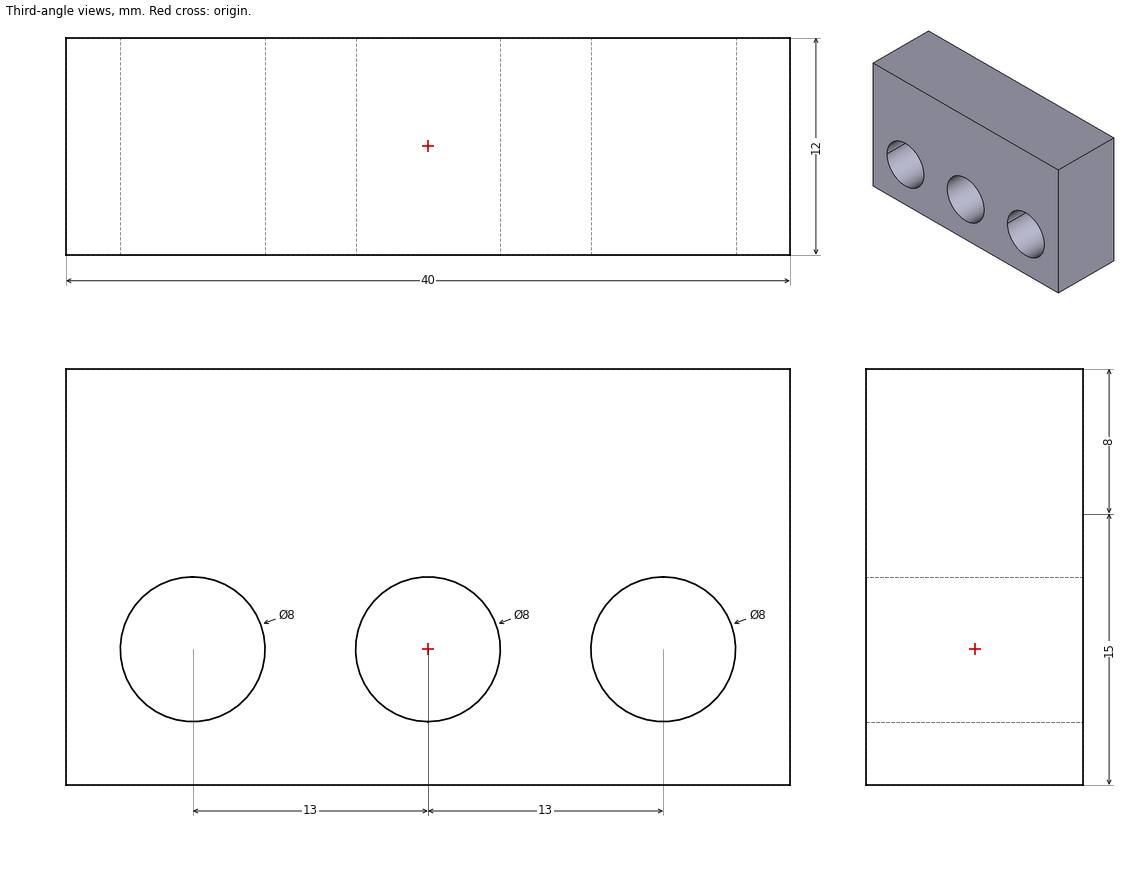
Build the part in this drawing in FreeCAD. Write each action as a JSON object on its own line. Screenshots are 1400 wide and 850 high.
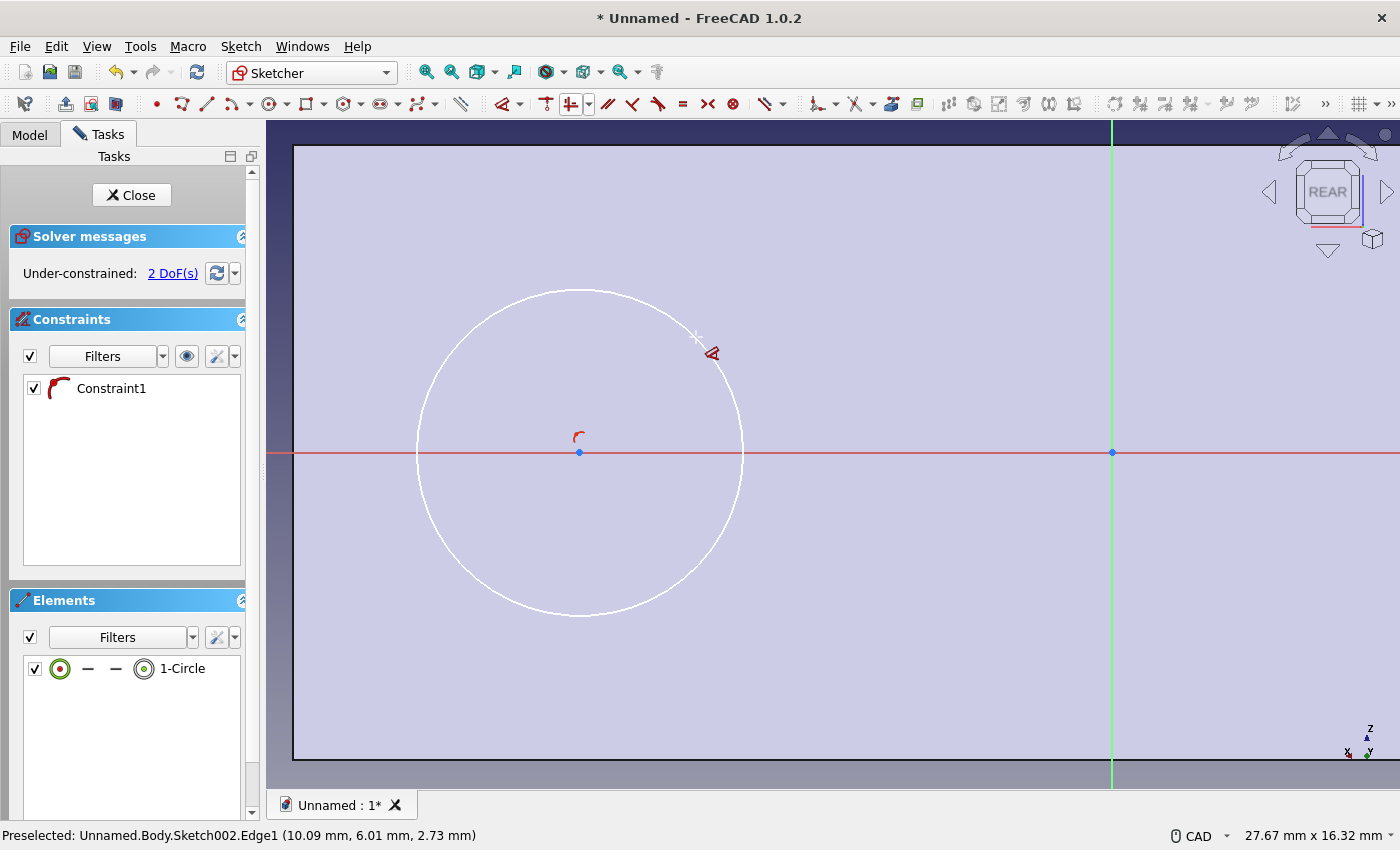
{"action": "left_click", "coordinate": [695, 337]}
{"action": "left_click", "coordinate": [718, 314]}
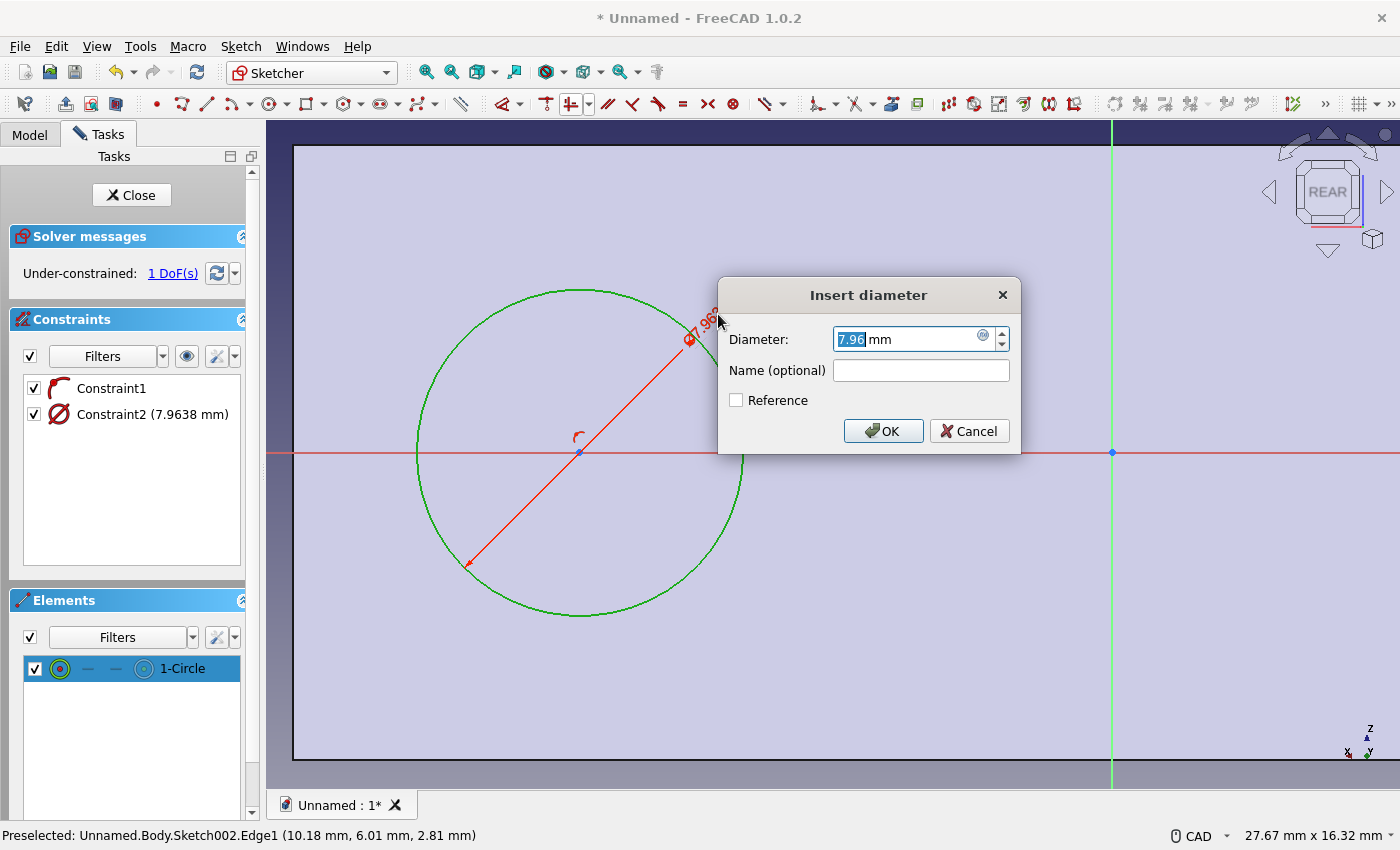
{"action": "type", "text": "8"}
{"action": "key", "text": "Return"}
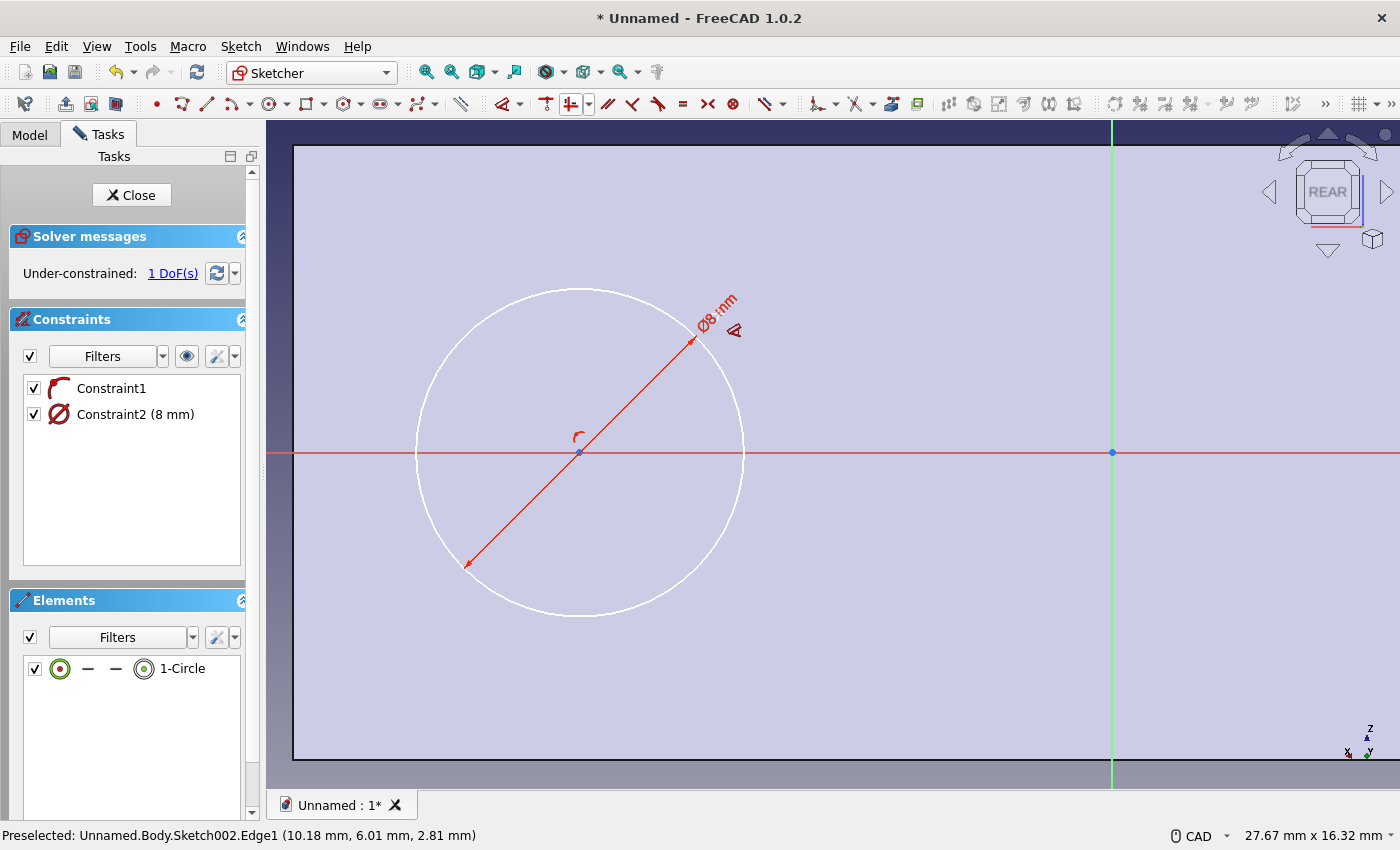
{"action": "left_click", "coordinate": [580, 453]}
{"action": "left_click", "coordinate": [846, 487]}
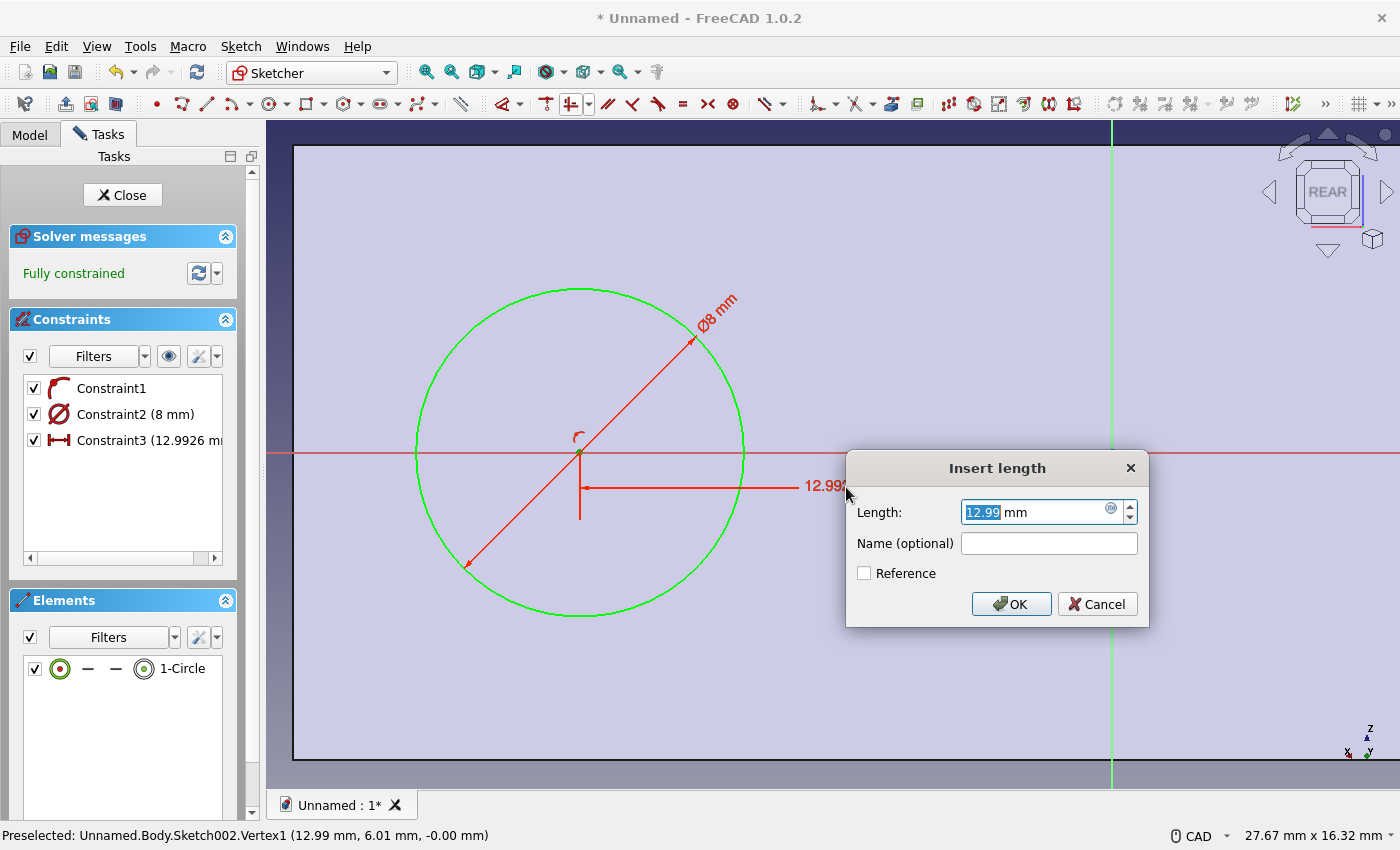
{"action": "type", "text": "13"}
{"action": "key", "text": "Return"}
{"action": "key", "text": "Escape"}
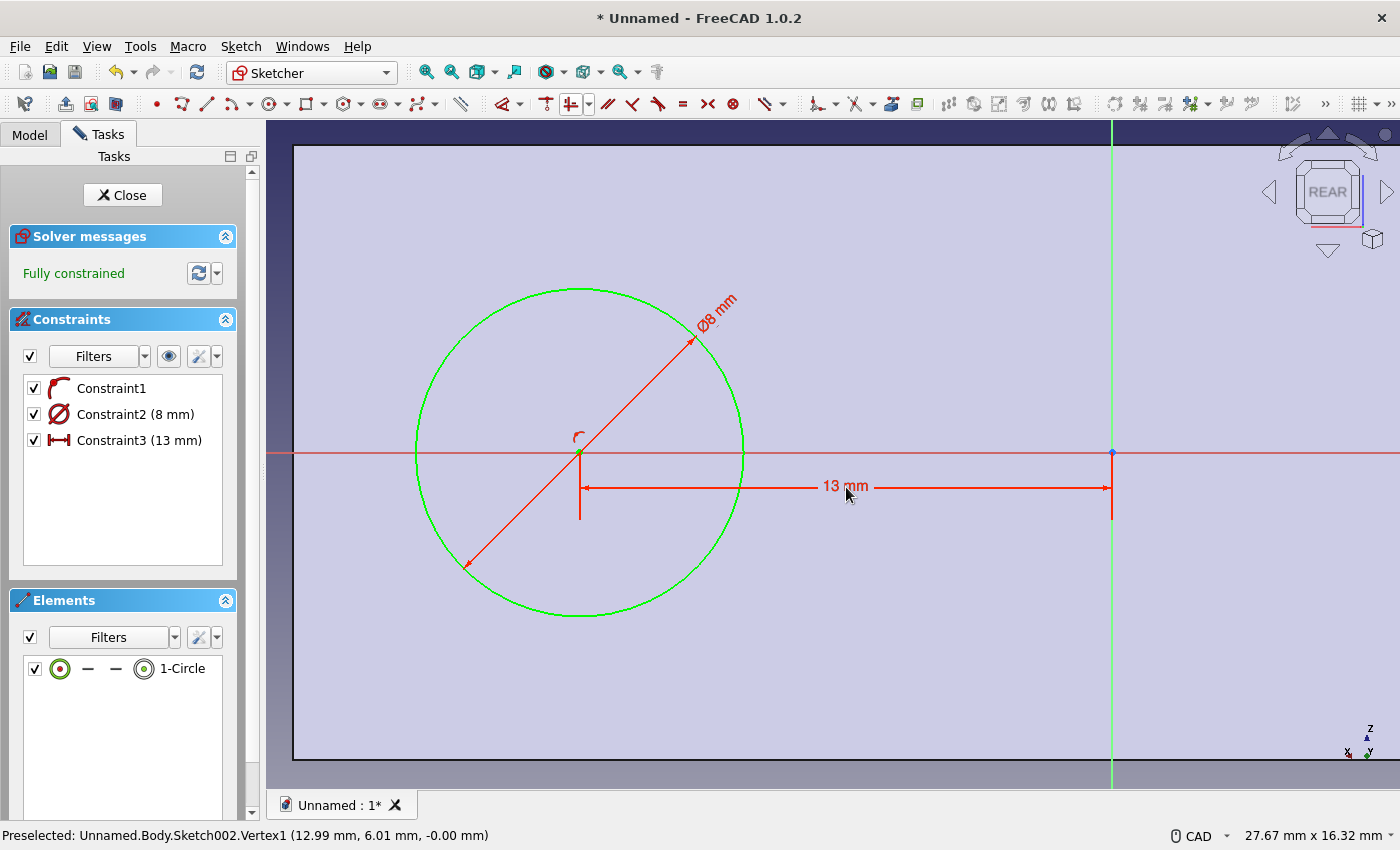
{"action": "left_click", "coordinate": [123, 195]}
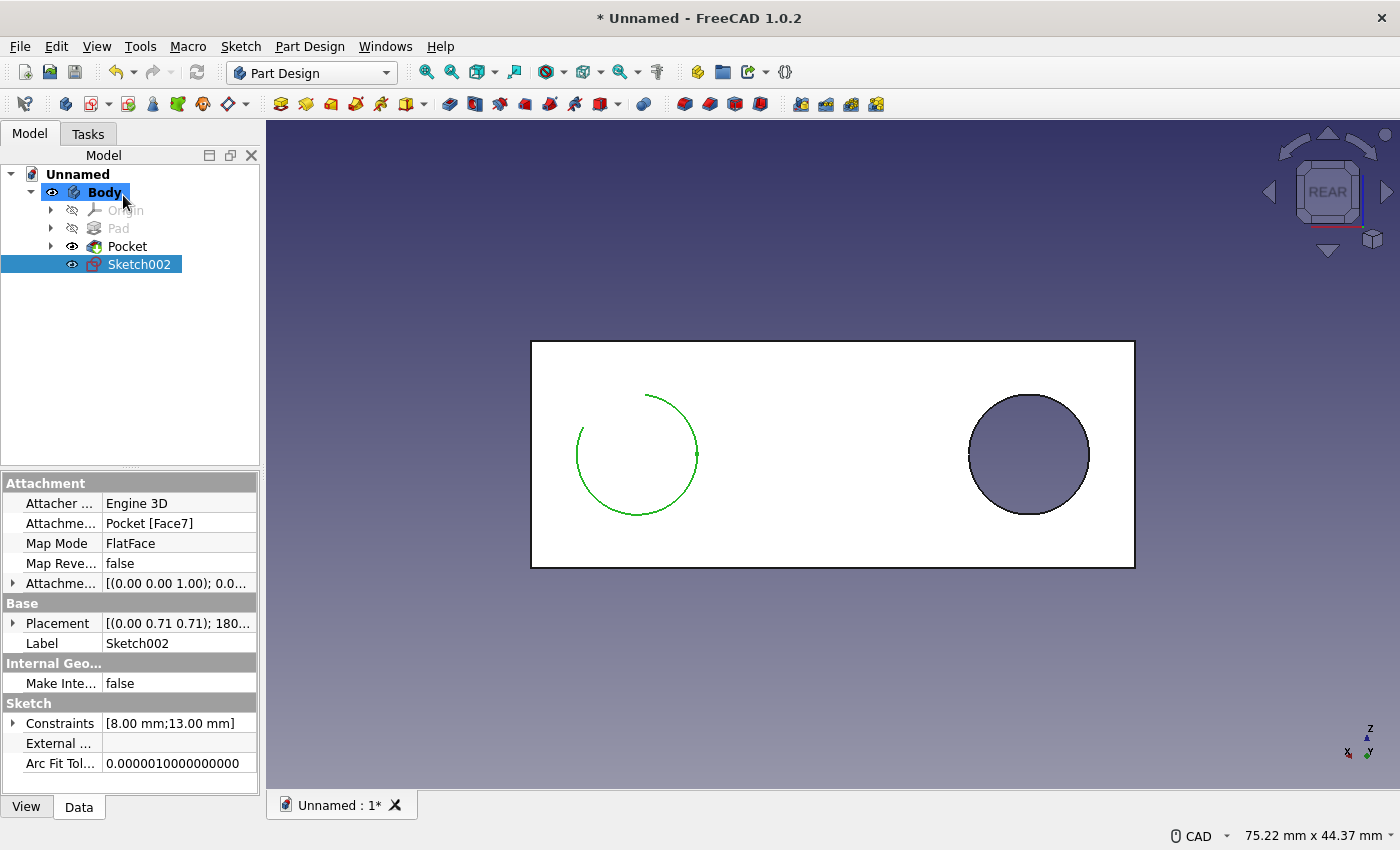
{"action": "left_click", "coordinate": [450, 104]}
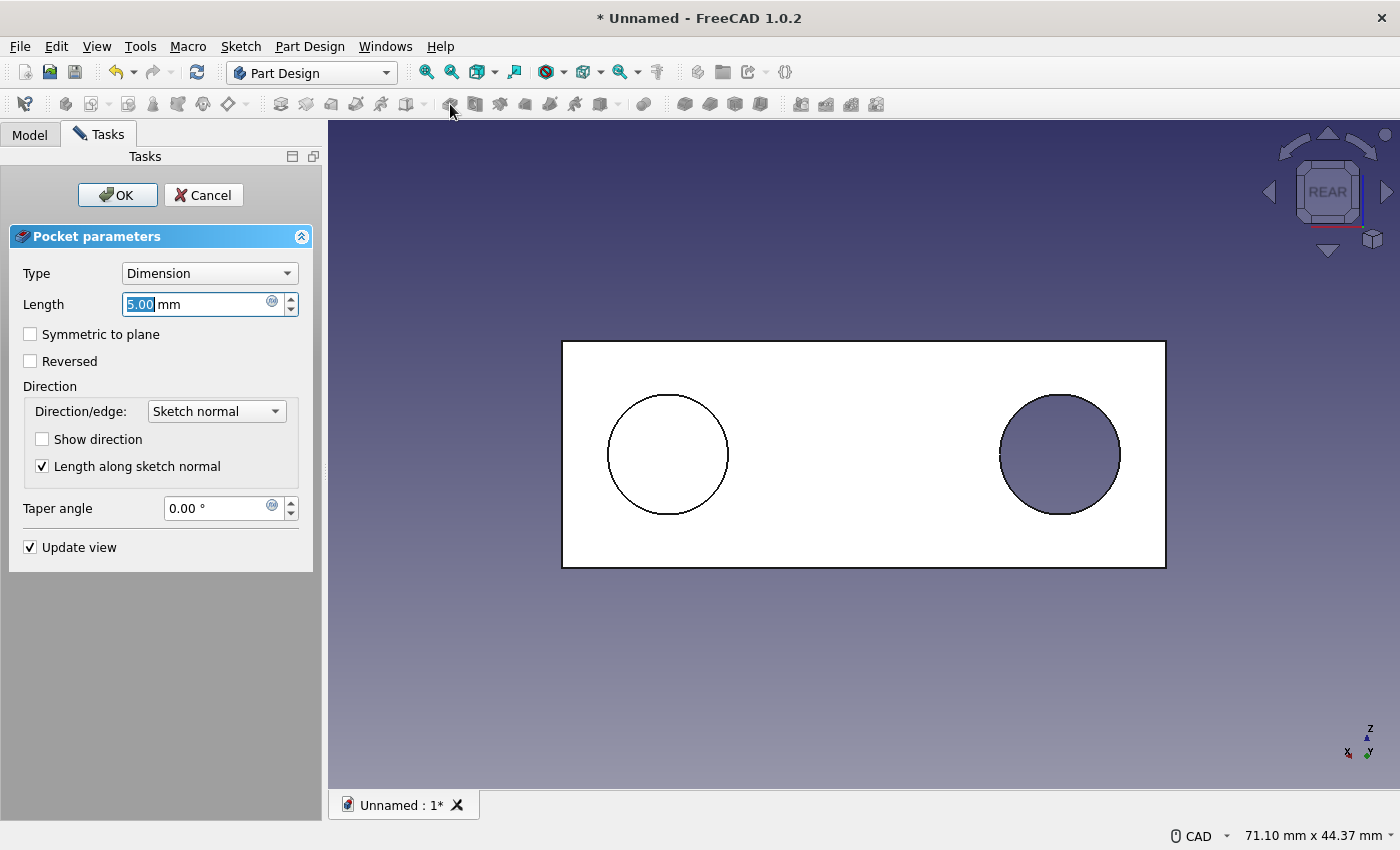
{"action": "left_click", "coordinate": [210, 274]}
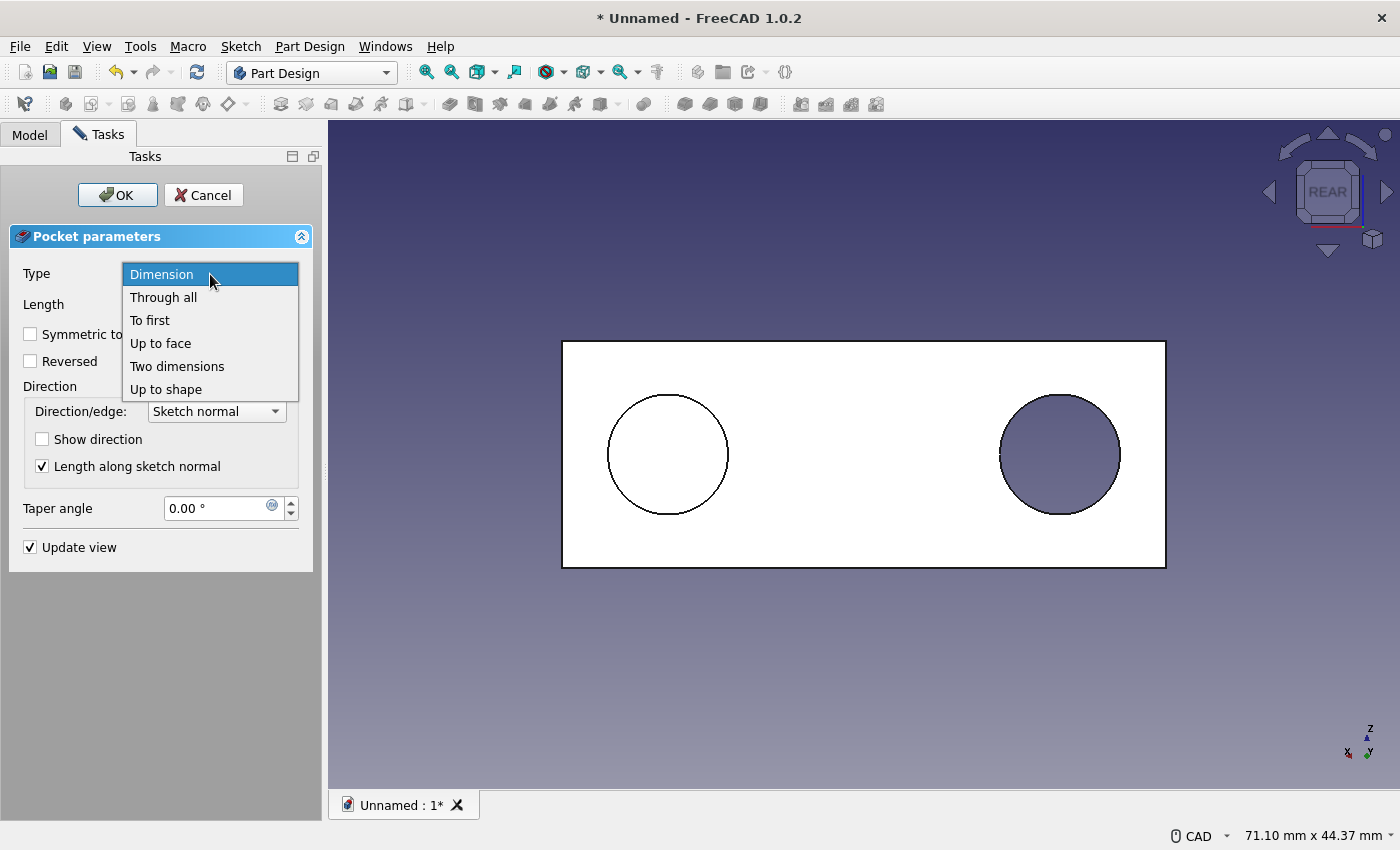
{"action": "left_click", "coordinate": [208, 320]}